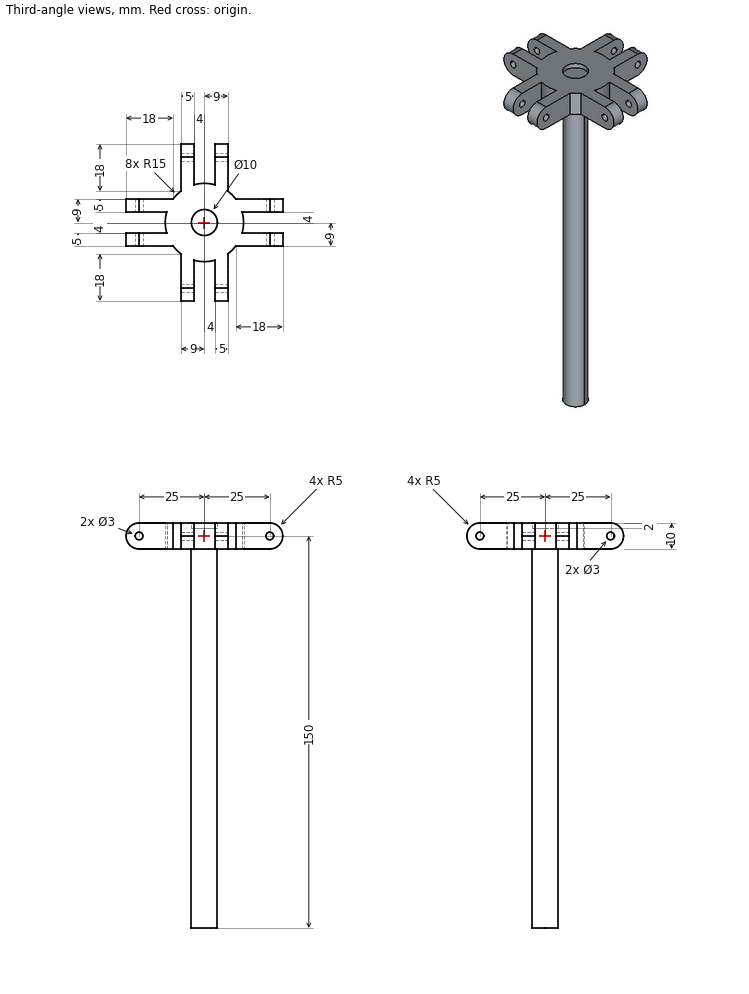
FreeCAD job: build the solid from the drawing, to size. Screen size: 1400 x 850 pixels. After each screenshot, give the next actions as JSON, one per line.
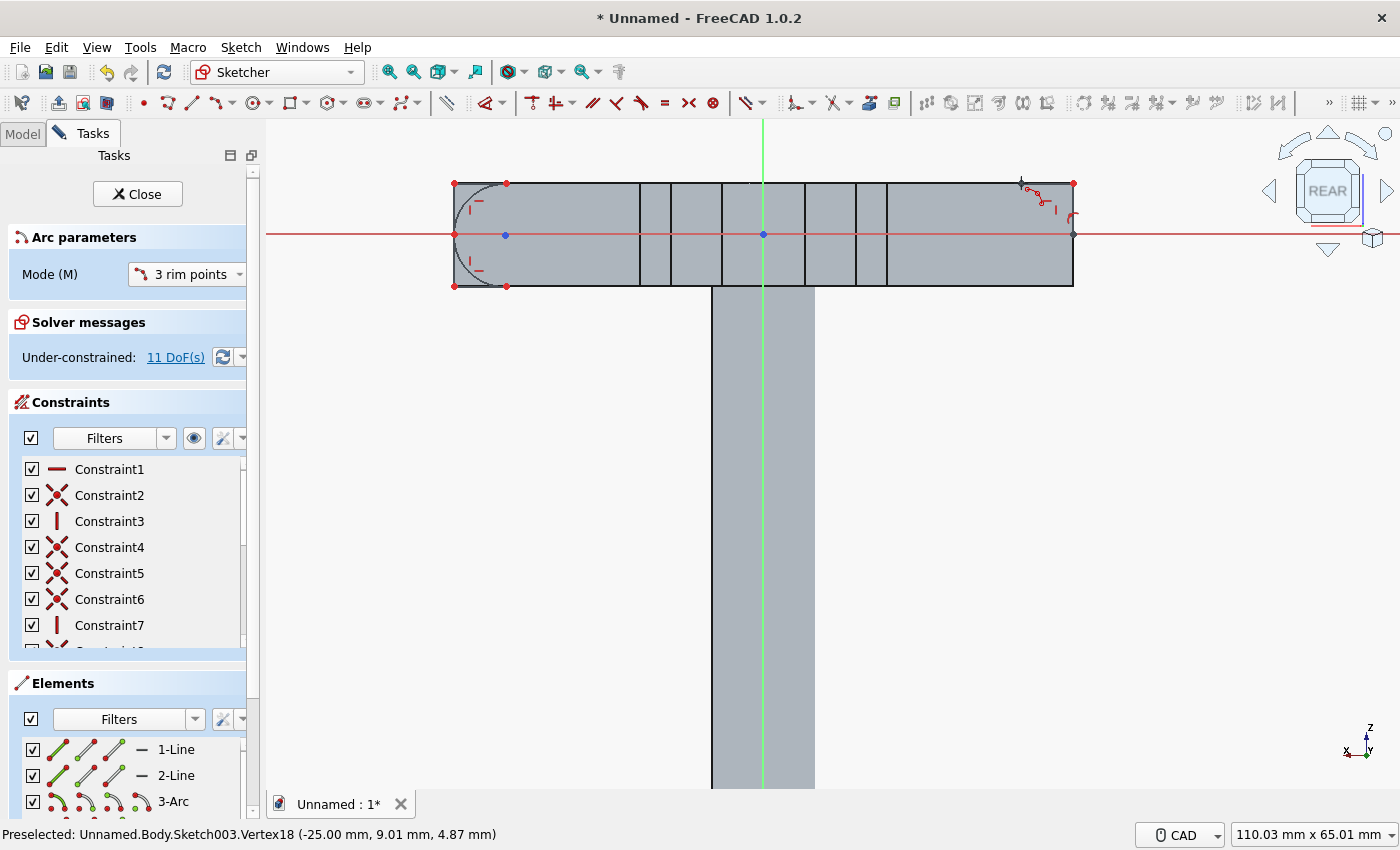
{"action": "left_click", "coordinate": [1021, 184]}
{"action": "left_click", "coordinate": [1073, 234]}
{"action": "left_click", "coordinate": [1057, 198]}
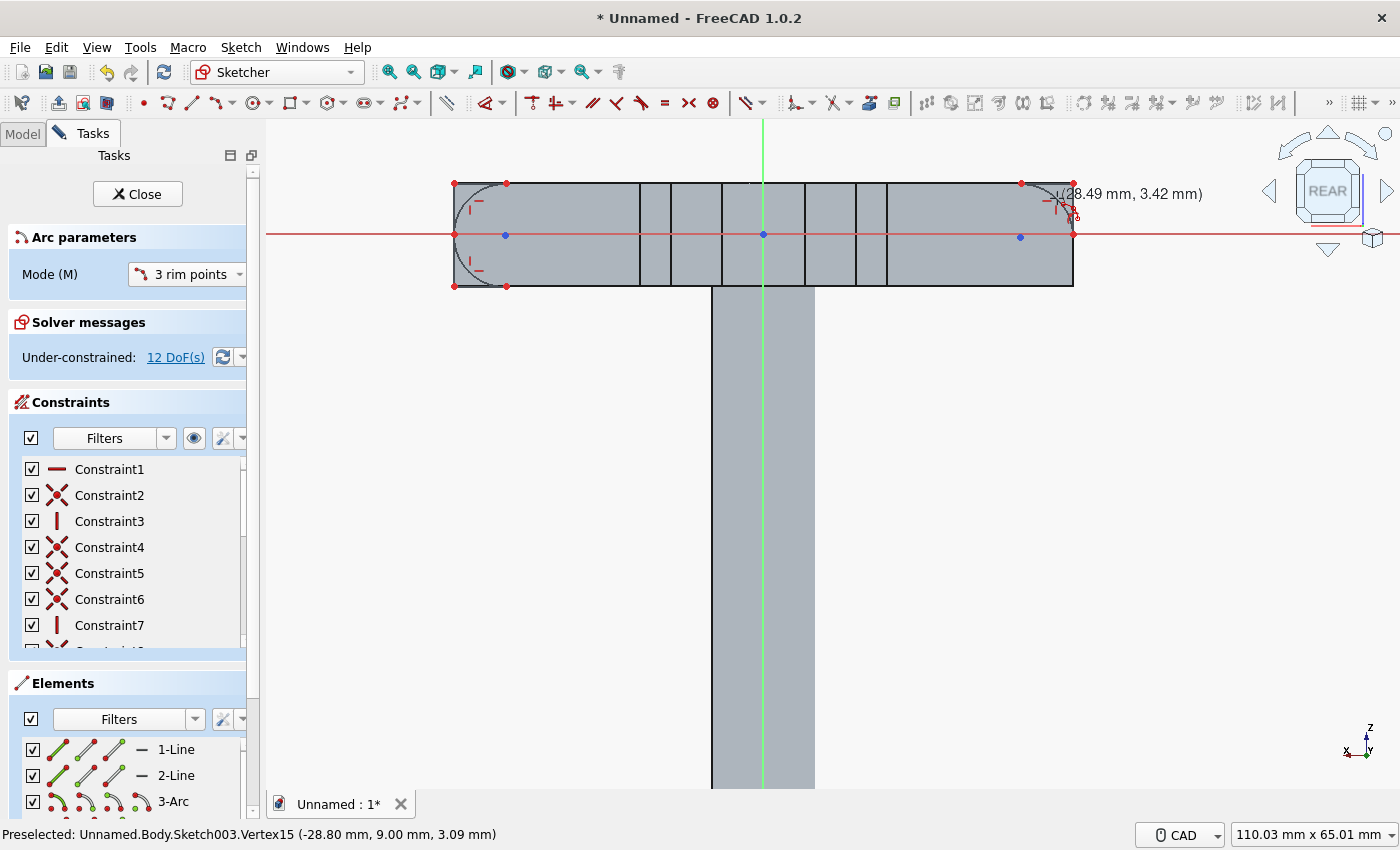
{"action": "left_click", "coordinate": [168, 104]}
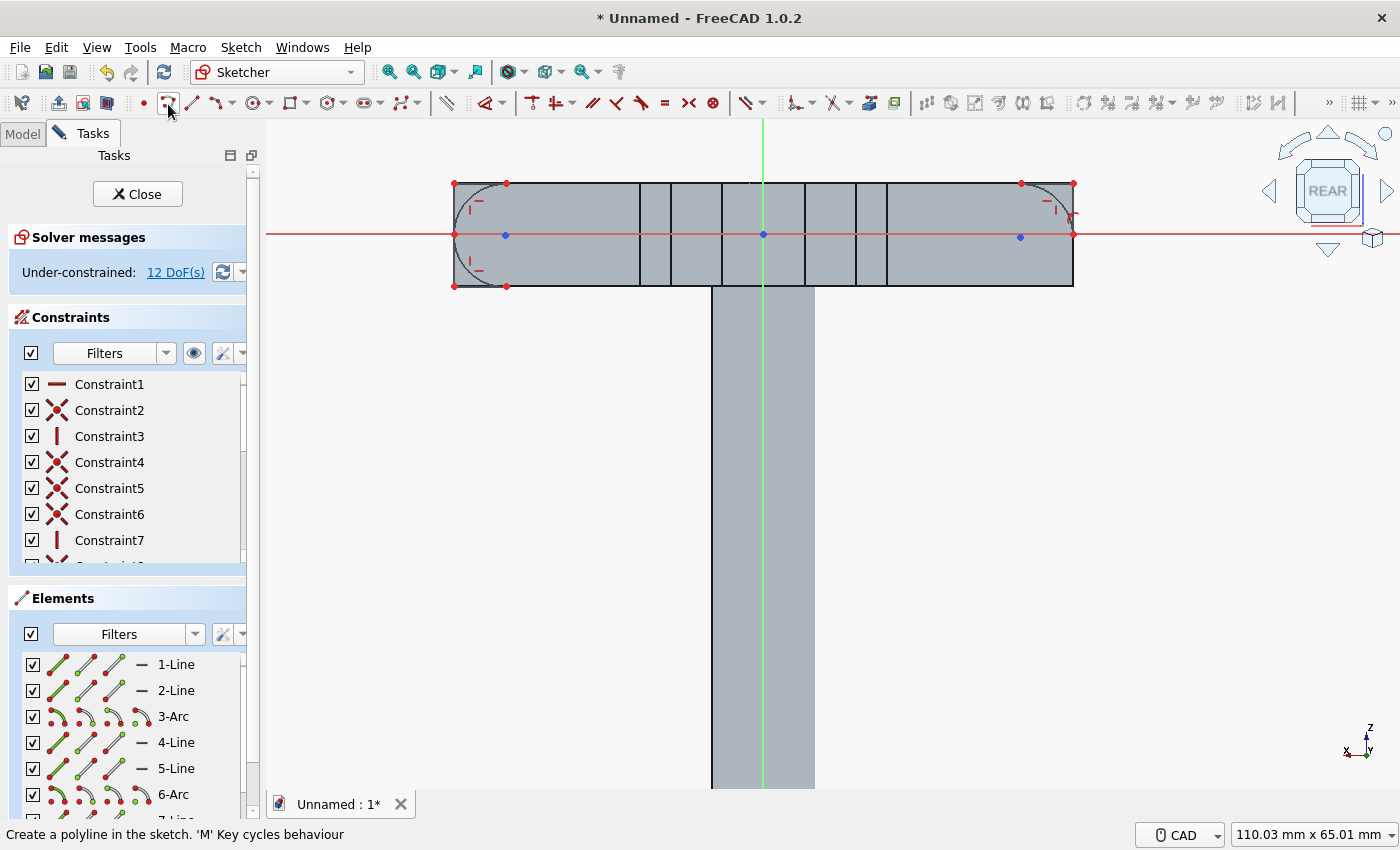
{"action": "left_click", "coordinate": [1021, 286]}
{"action": "left_click", "coordinate": [1073, 286]}
{"action": "left_click", "coordinate": [1073, 234]}
{"action": "right_click", "coordinate": [1073, 286]}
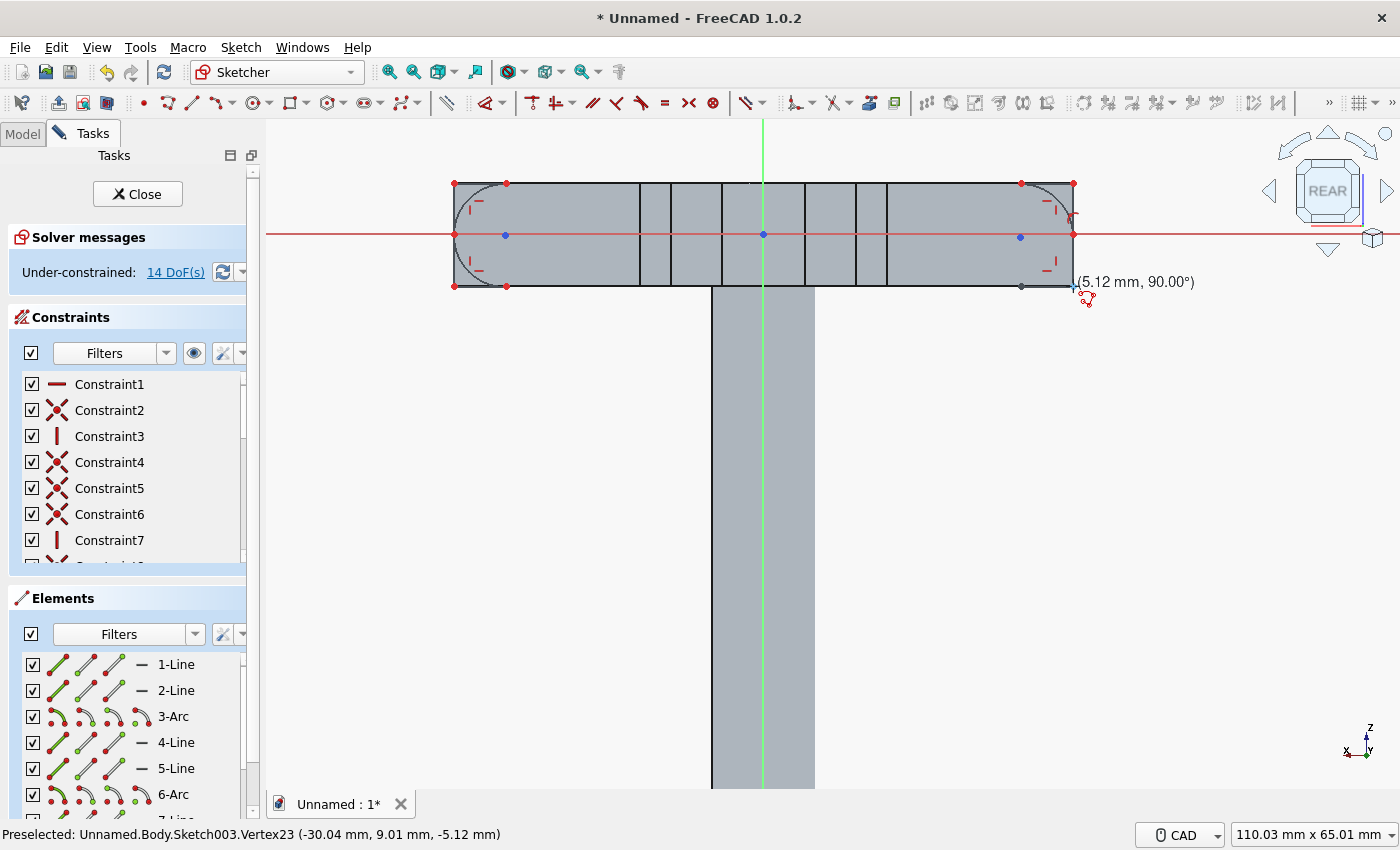
{"action": "left_click", "coordinate": [216, 104]}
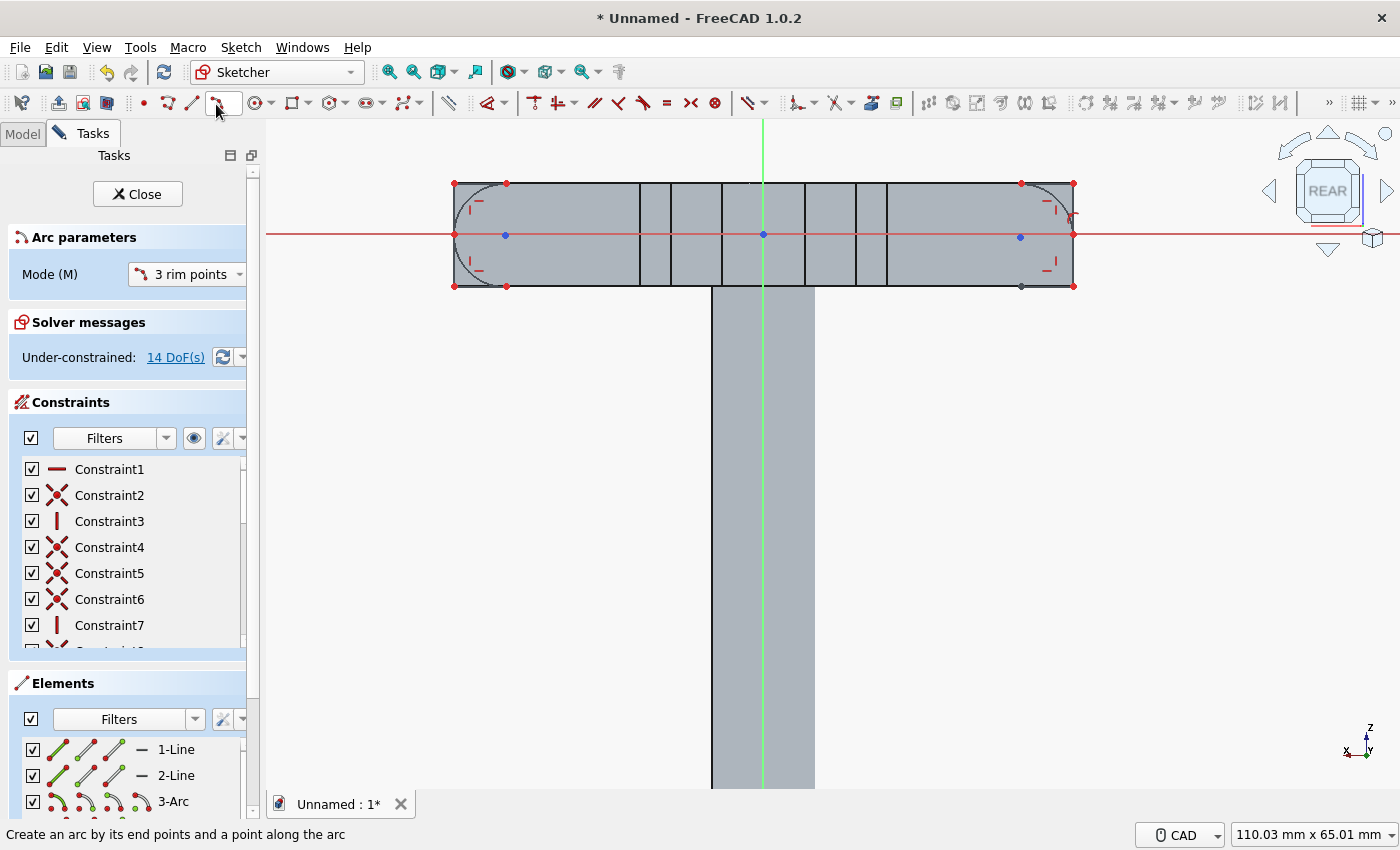
{"action": "left_click", "coordinate": [1073, 234]}
{"action": "left_click", "coordinate": [1021, 287]}
{"action": "left_click", "coordinate": [1057, 271]}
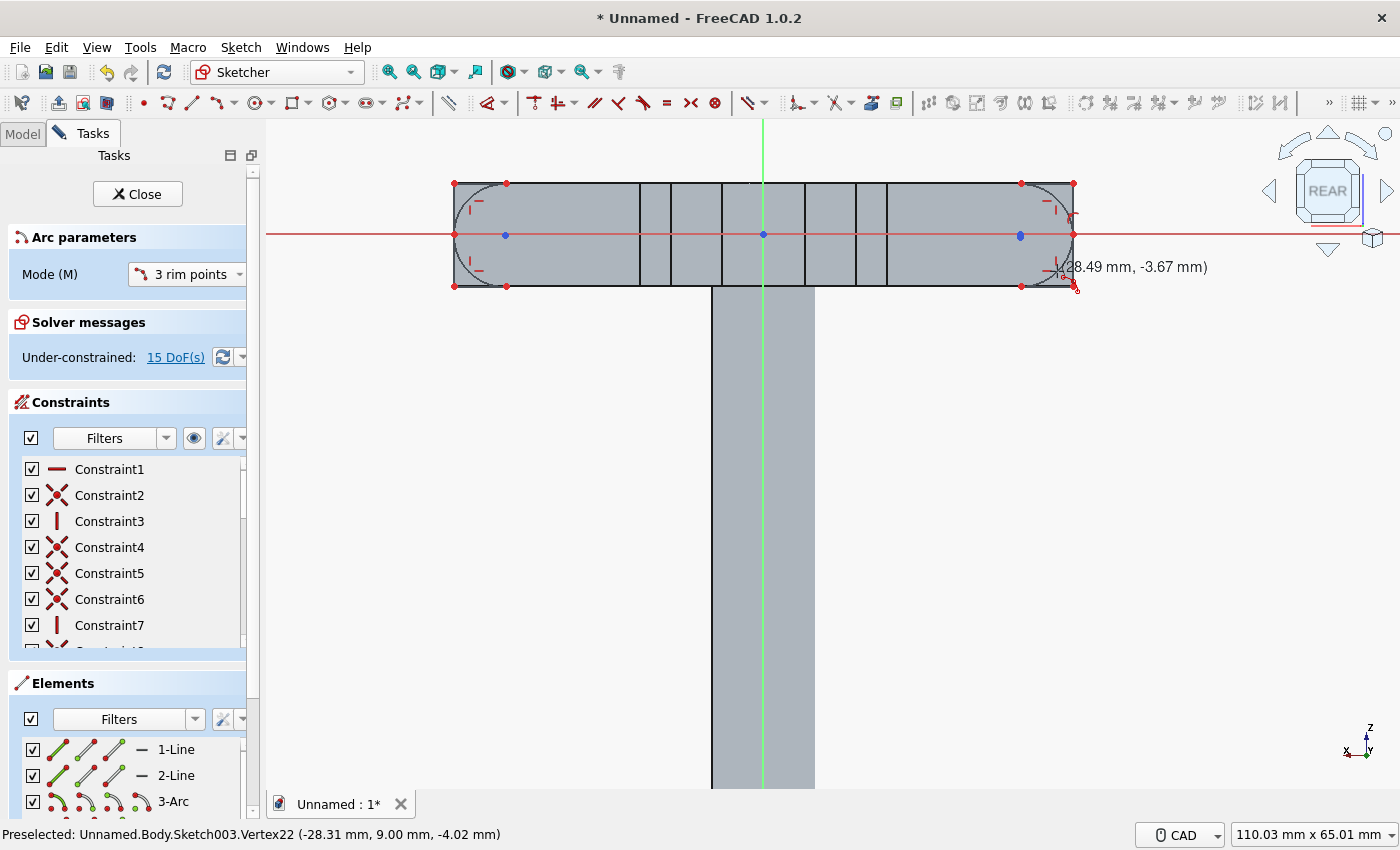
{"action": "left_click", "coordinate": [256, 104]}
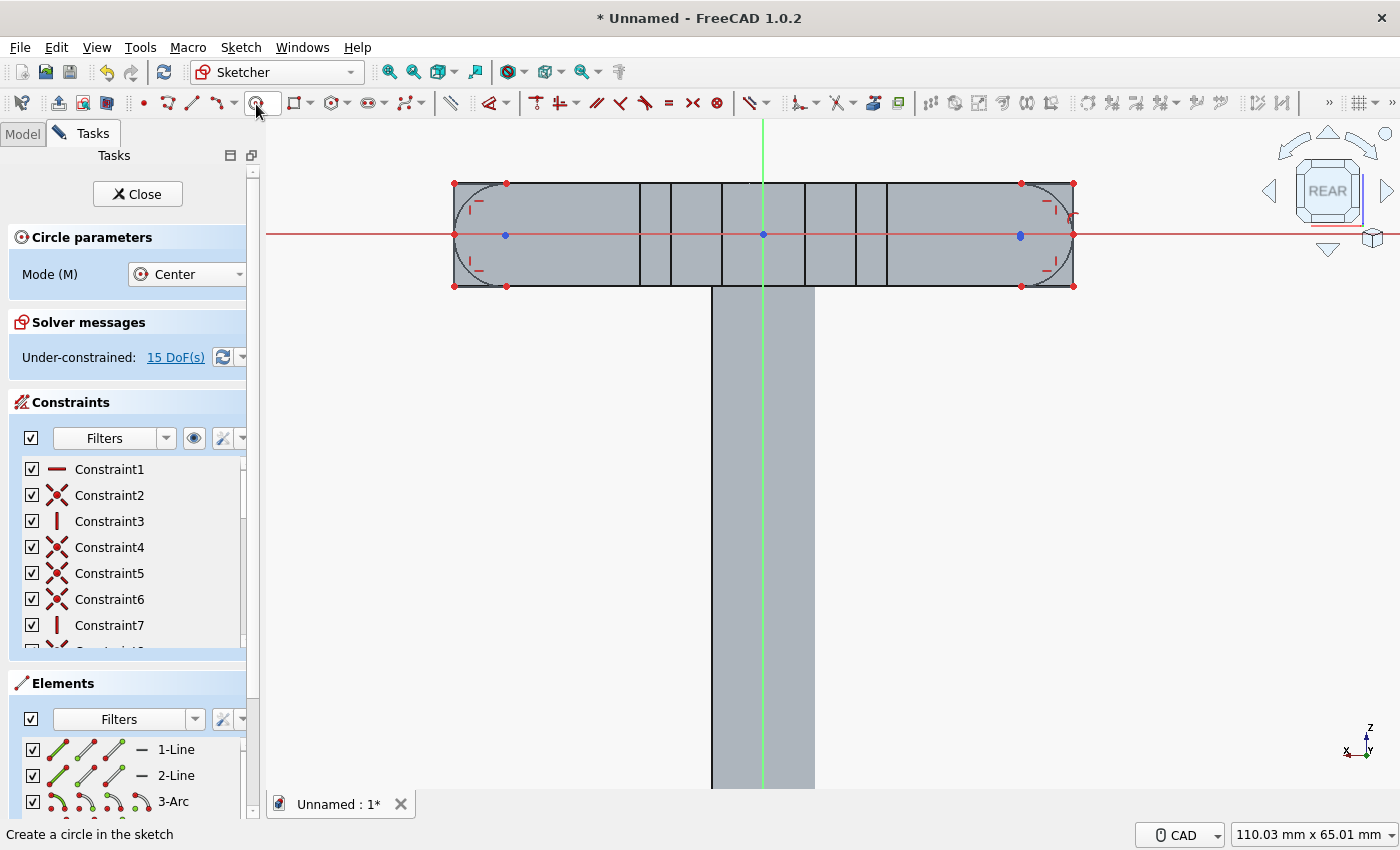
{"action": "scroll", "coordinate": [1021, 234], "scroll_direction": "up", "scroll_amount": 2}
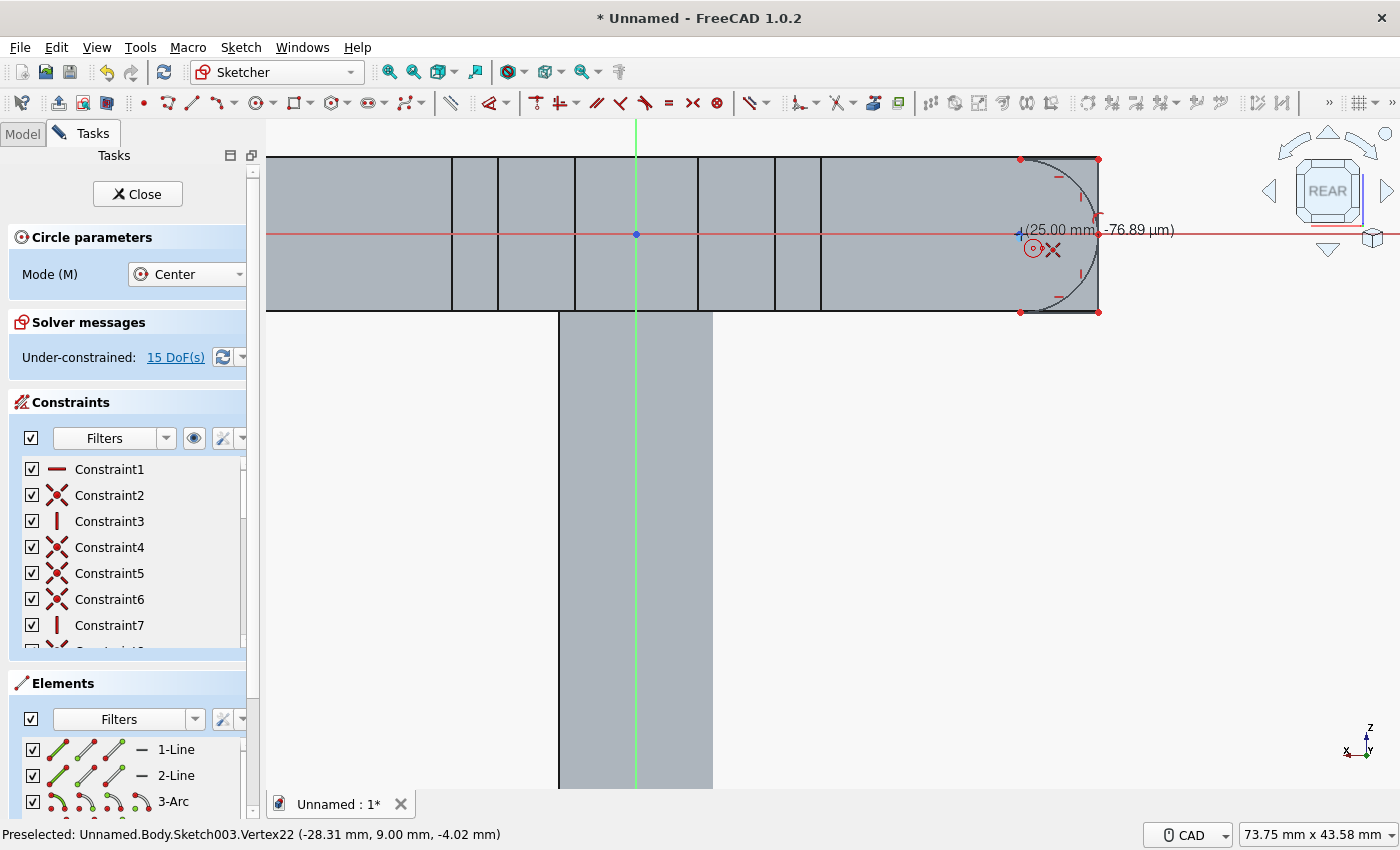
{"action": "left_click", "coordinate": [1021, 234]}
{"action": "mouse_move", "coordinate": [1037, 218]}